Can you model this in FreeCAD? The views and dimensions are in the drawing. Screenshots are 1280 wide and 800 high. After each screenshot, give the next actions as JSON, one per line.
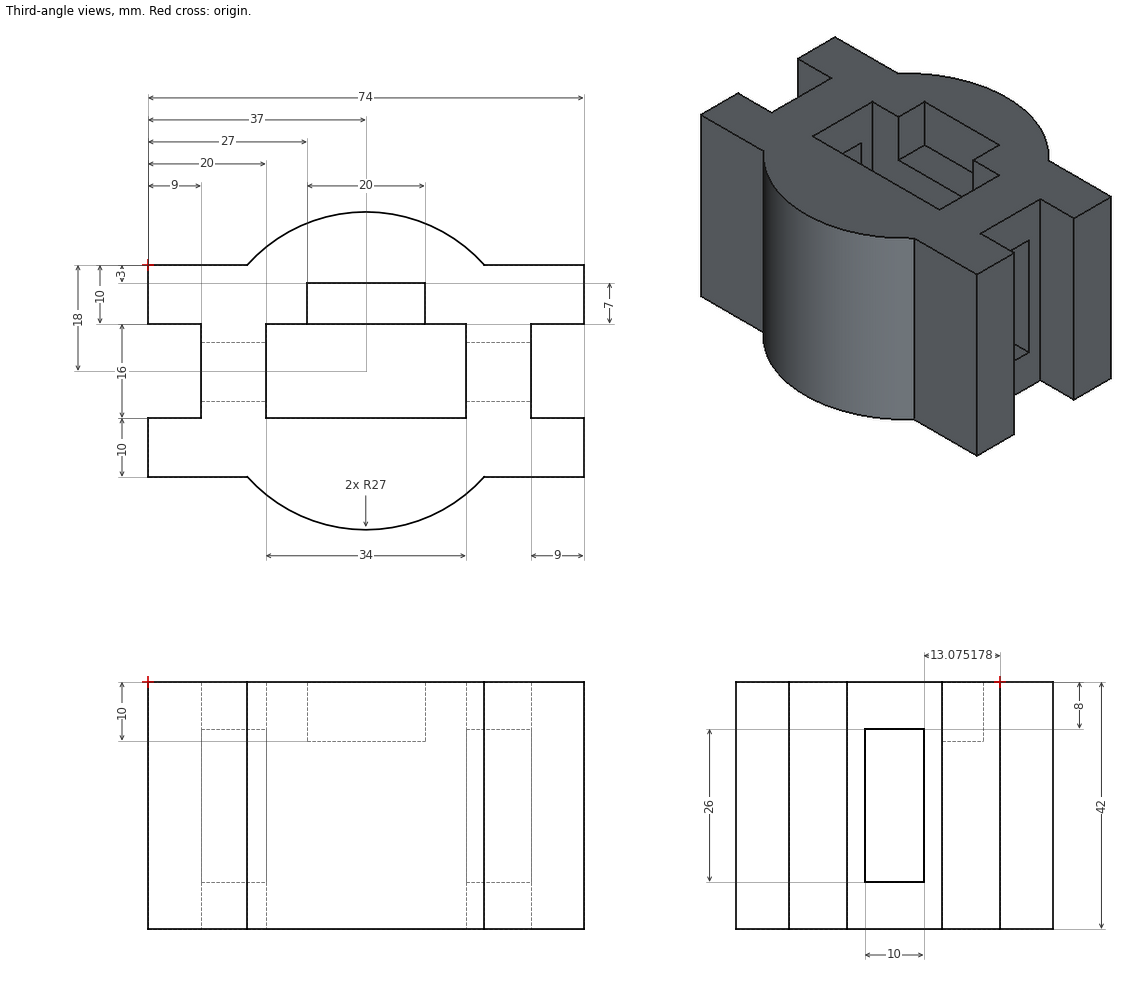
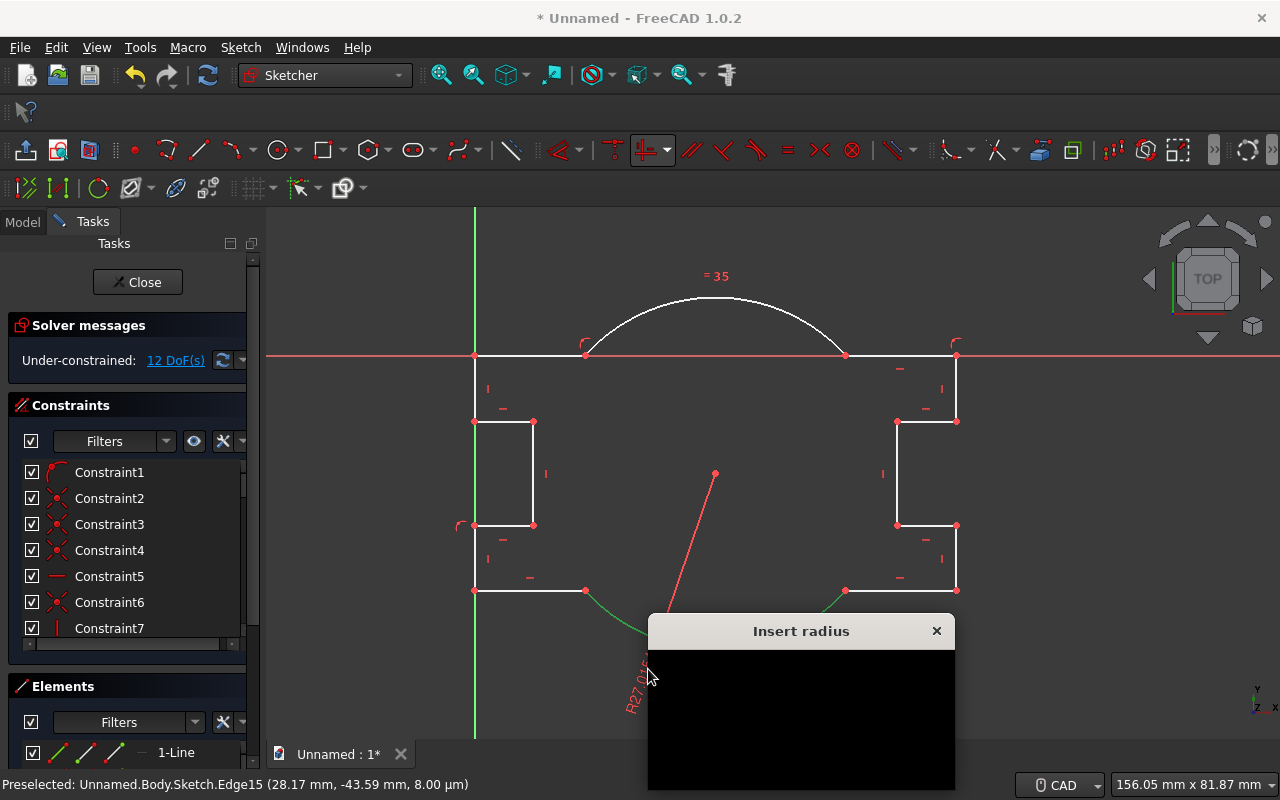
{"action": "type", "text": "27"}
{"action": "key", "text": "Return"}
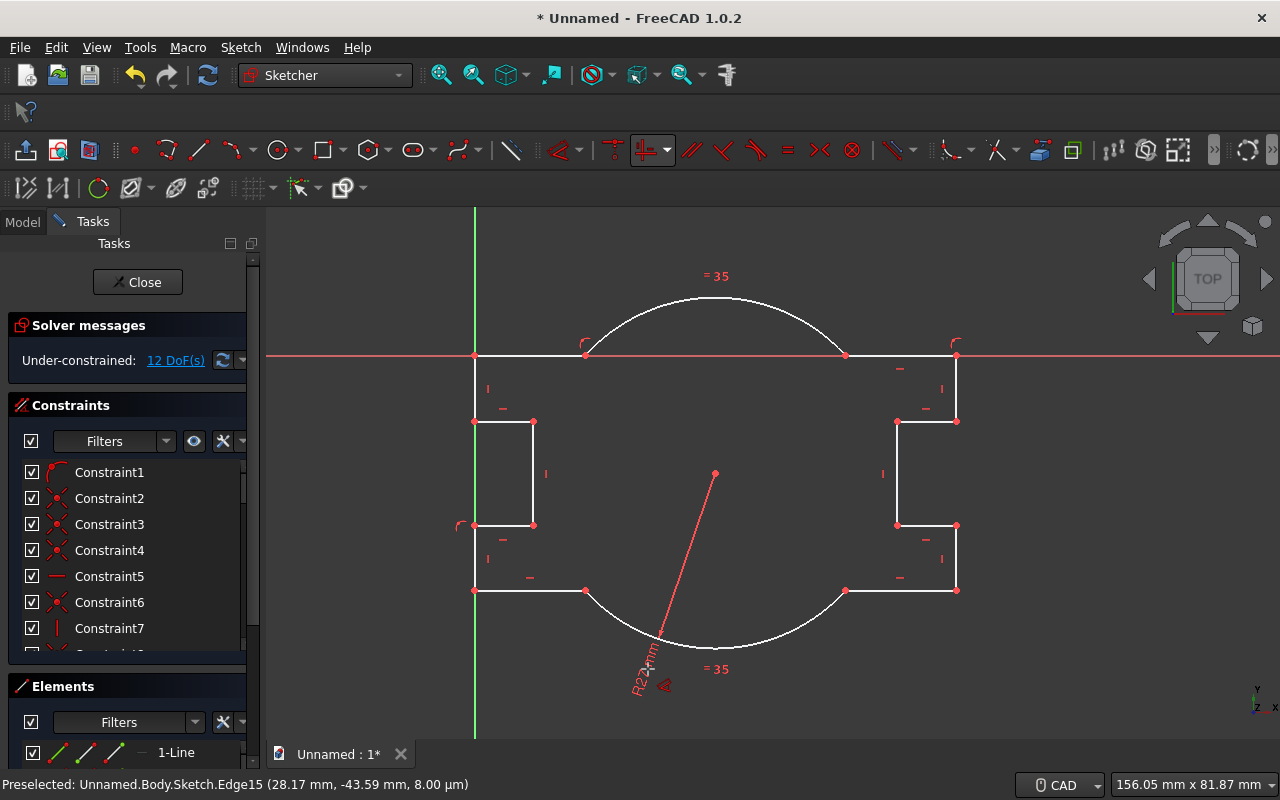
{"action": "left_click", "coordinate": [492, 422]}
{"action": "left_click", "coordinate": [504, 388]}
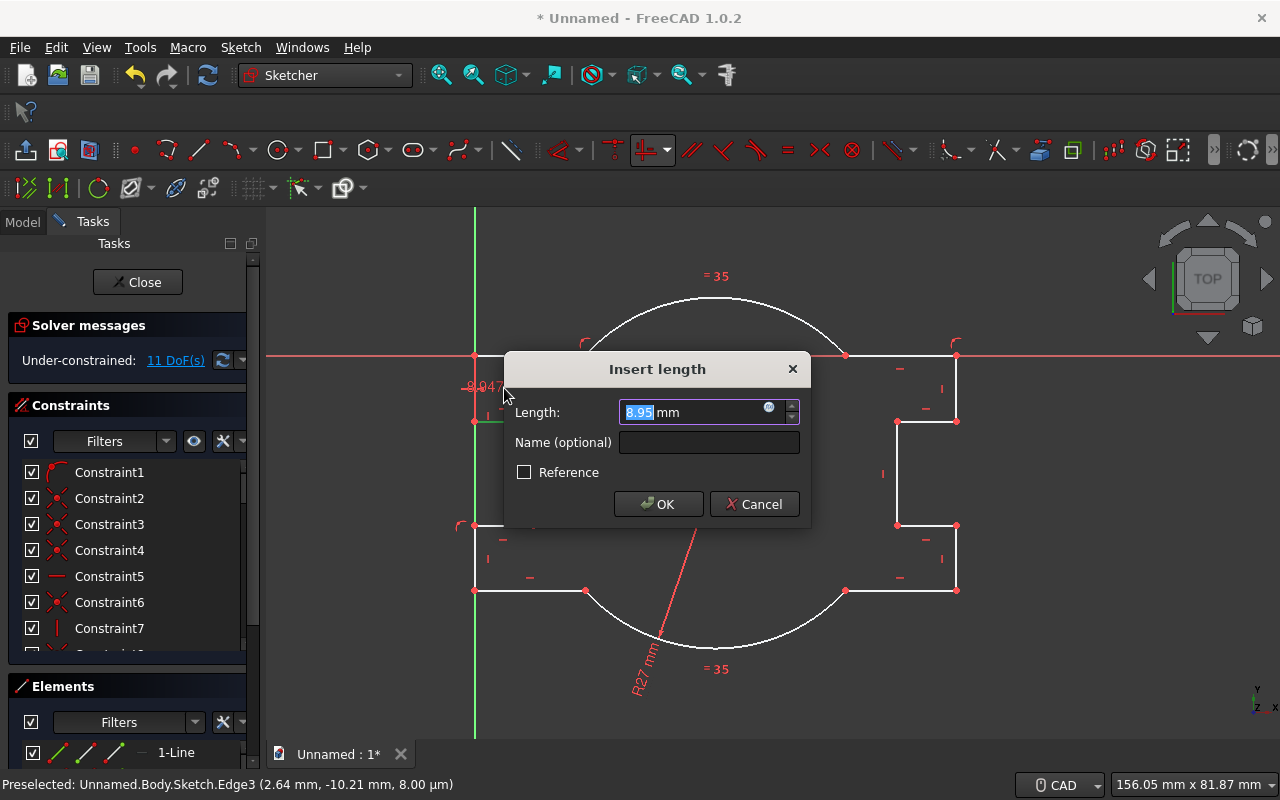
{"action": "type", "text": "9"}
{"action": "key", "text": "Return"}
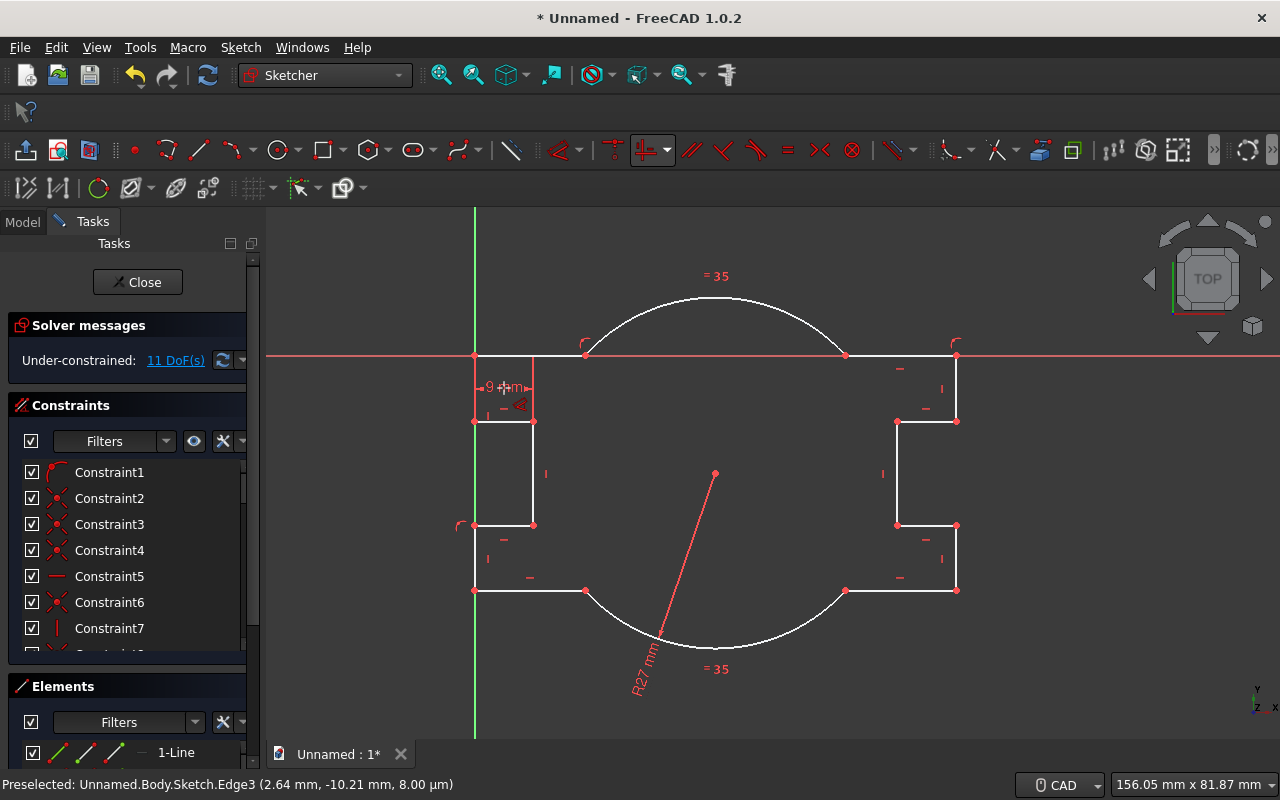
{"action": "left_click", "coordinate": [938, 526]}
{"action": "left_click", "coordinate": [927, 560]}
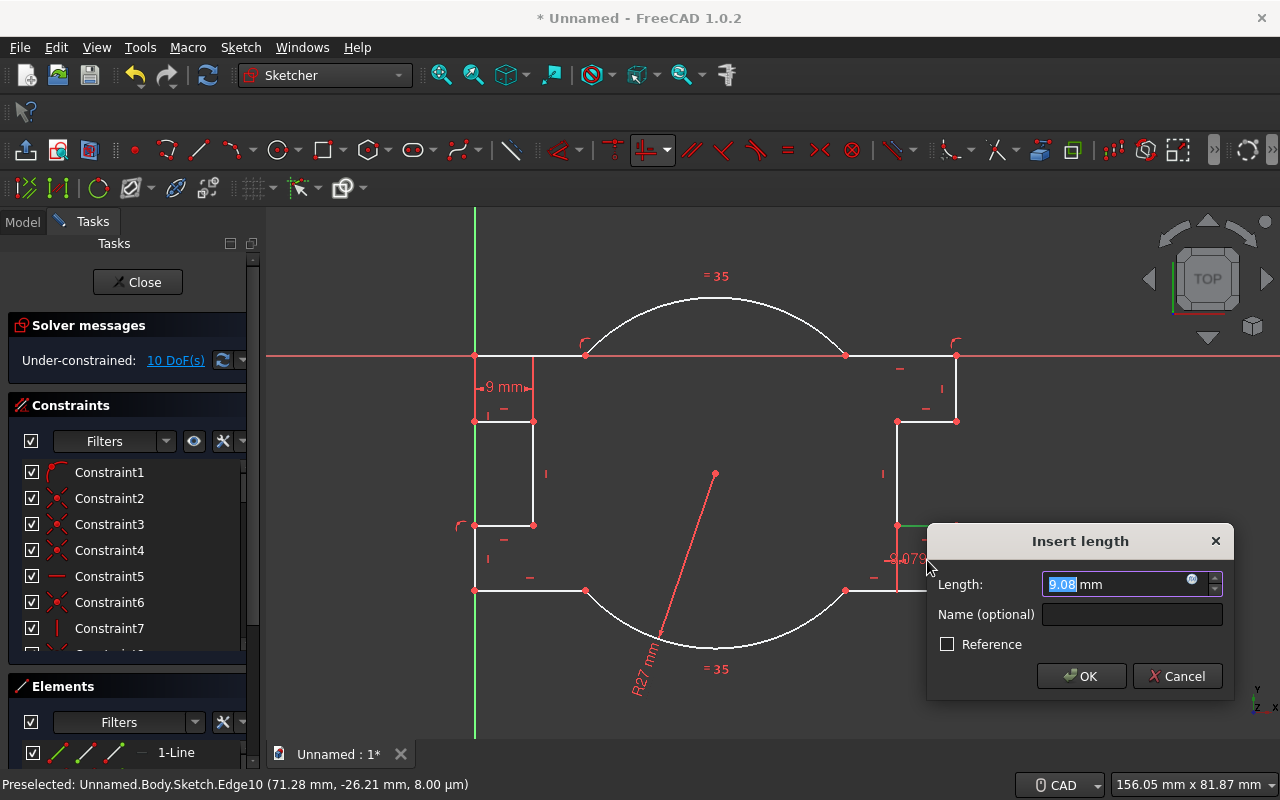
{"action": "type", "text": "9"}
{"action": "key", "text": "Return"}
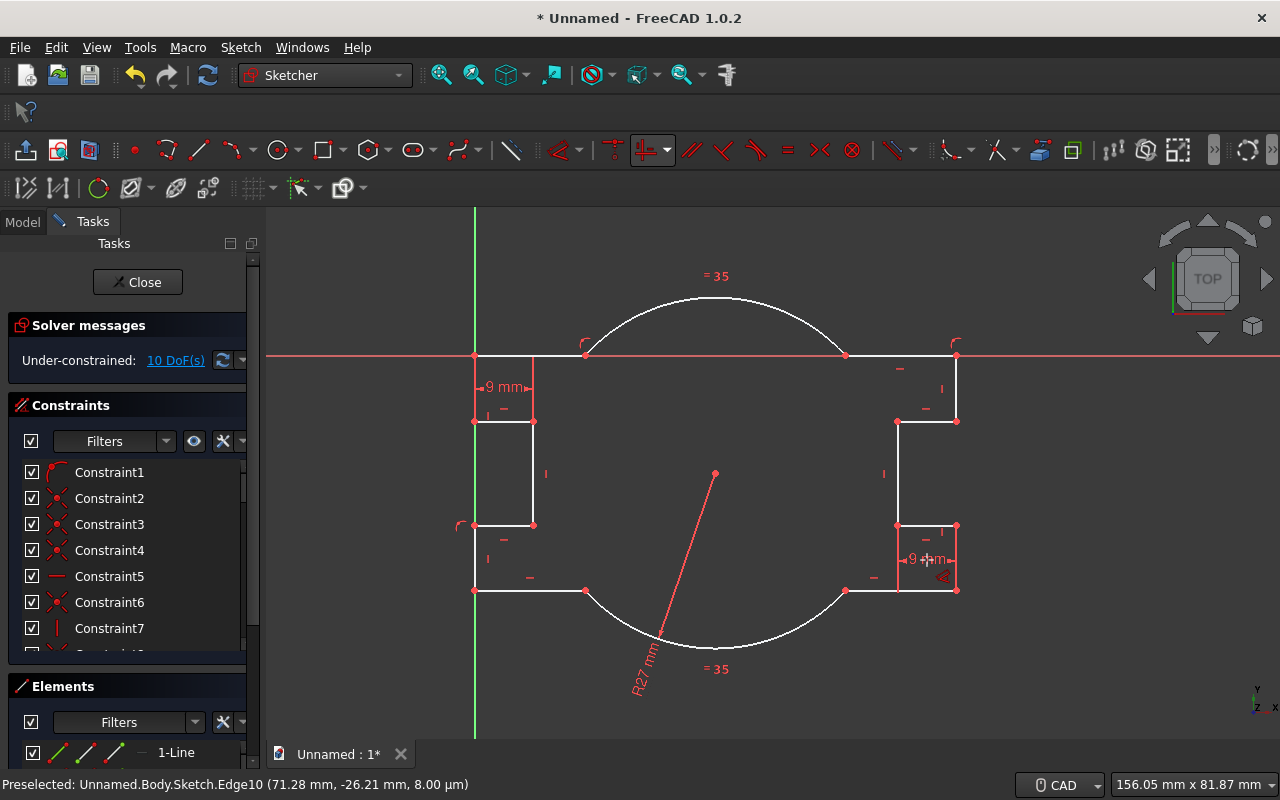
{"action": "left_click", "coordinate": [915, 422]}
{"action": "left_click", "coordinate": [927, 388]}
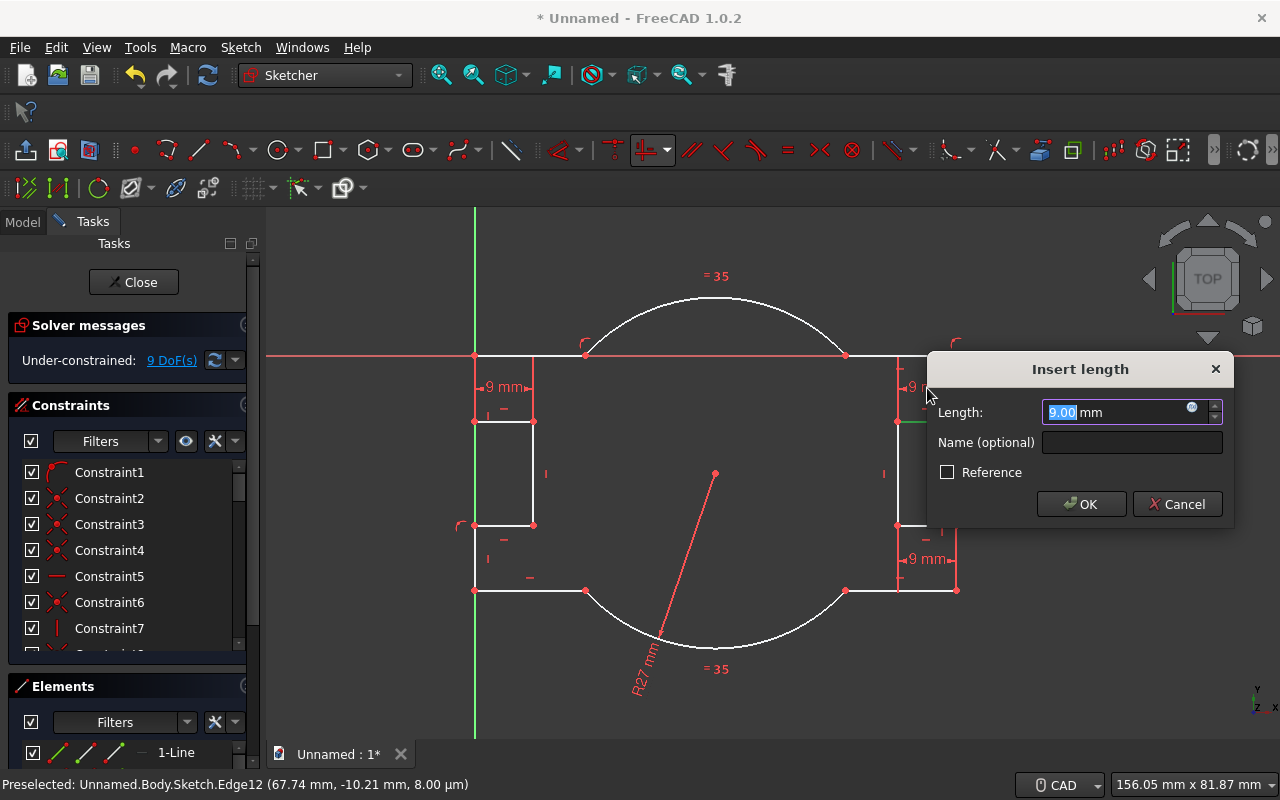
{"action": "type", "text": "9"}
{"action": "key", "text": "Return"}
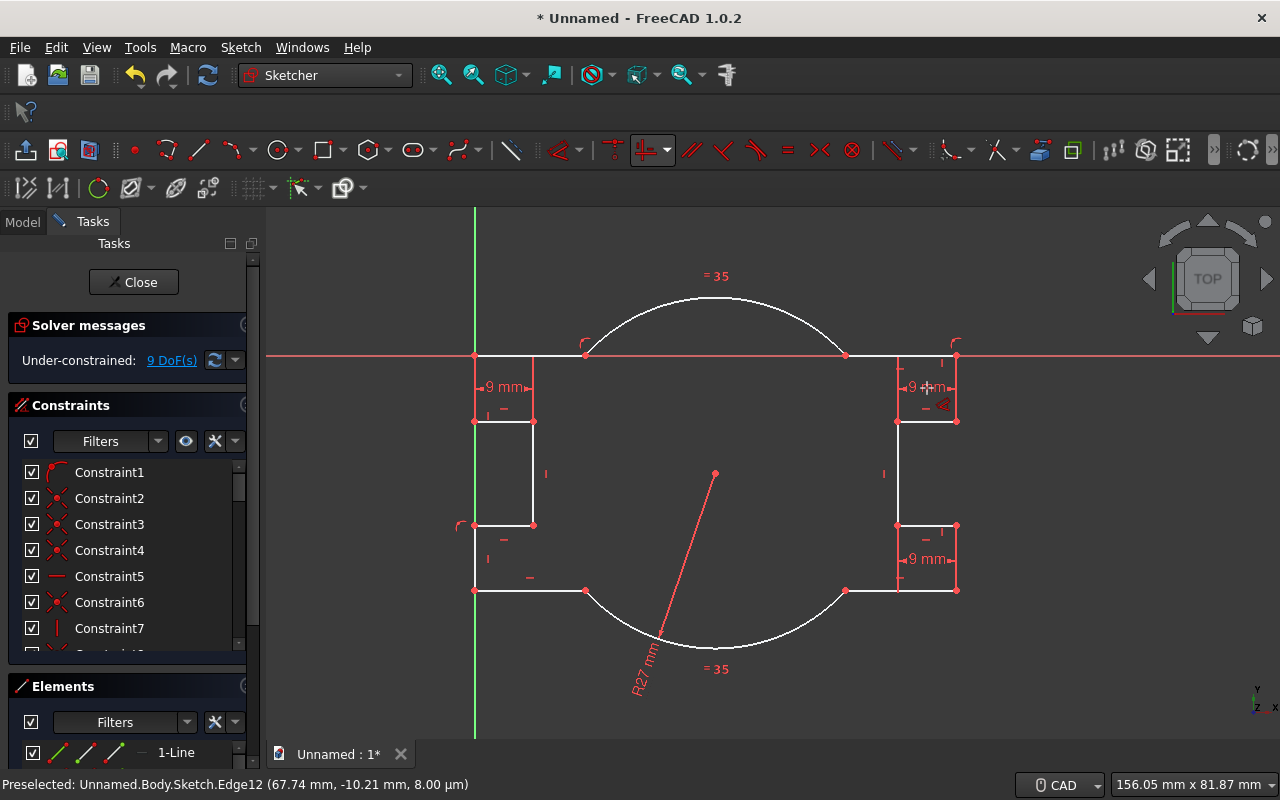
{"action": "left_click", "coordinate": [475, 376]}
{"action": "left_click", "coordinate": [441, 412]}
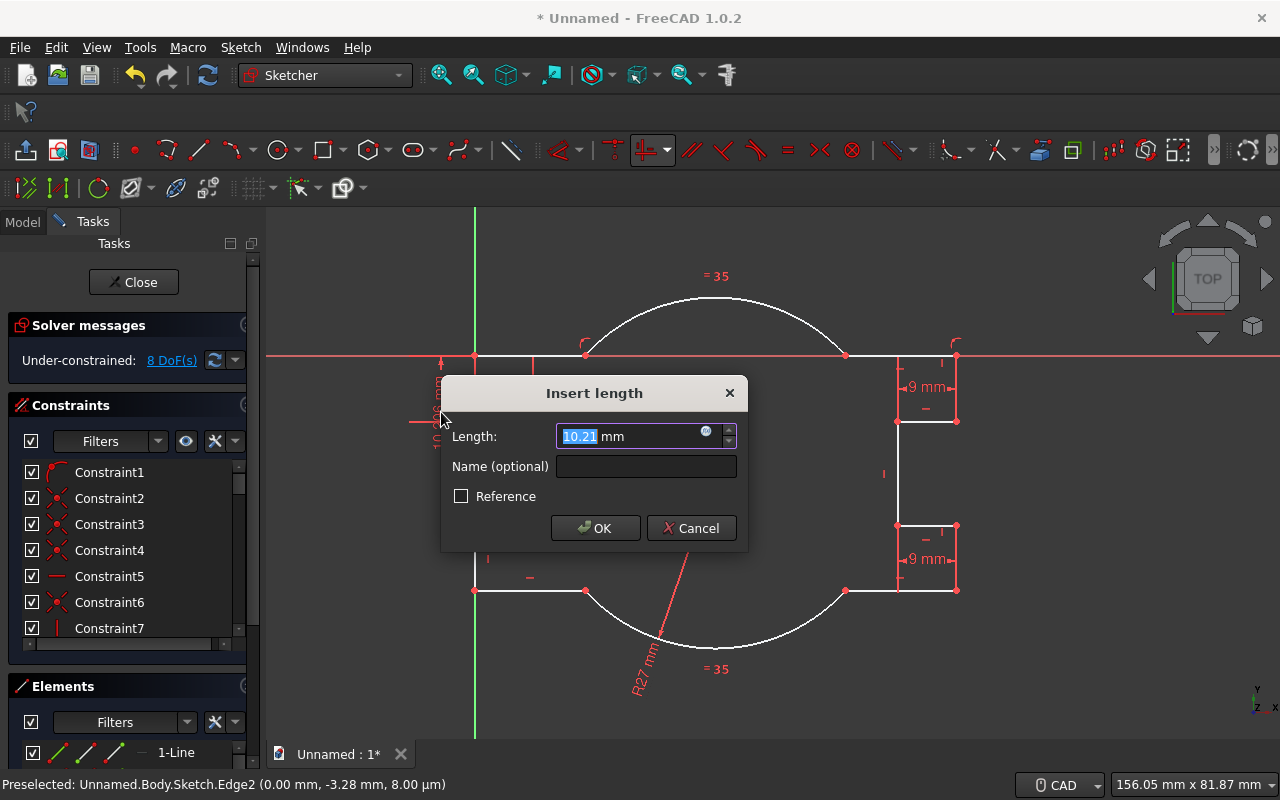
{"action": "type", "text": "10"}
{"action": "key", "text": "Return"}